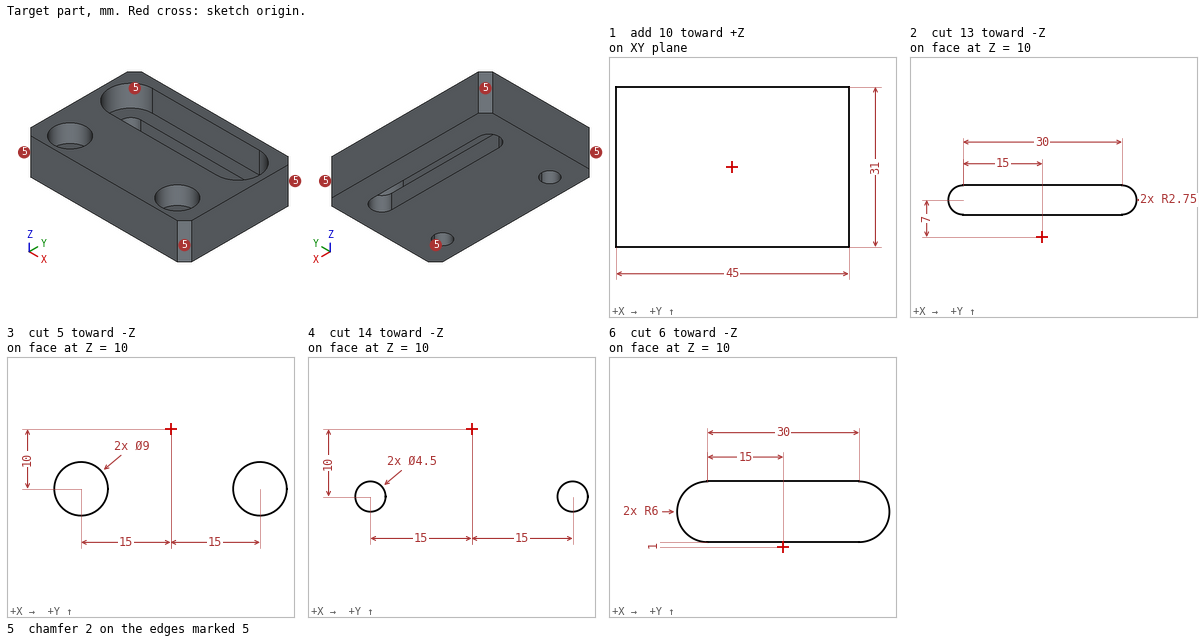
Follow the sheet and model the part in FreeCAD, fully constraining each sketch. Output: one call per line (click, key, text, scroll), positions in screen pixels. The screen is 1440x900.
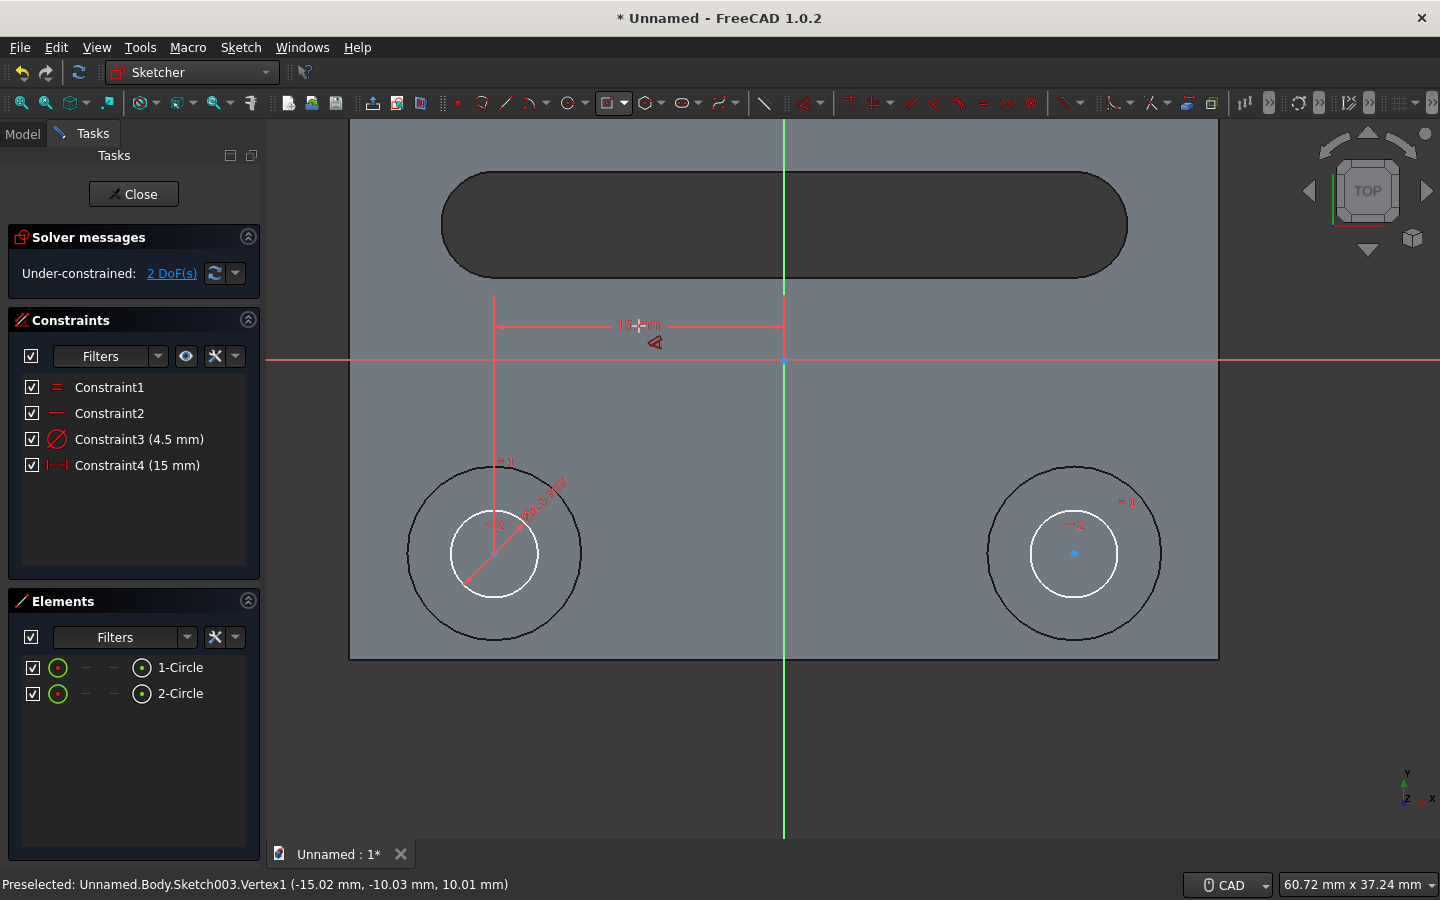
click(494, 554)
click(460, 457)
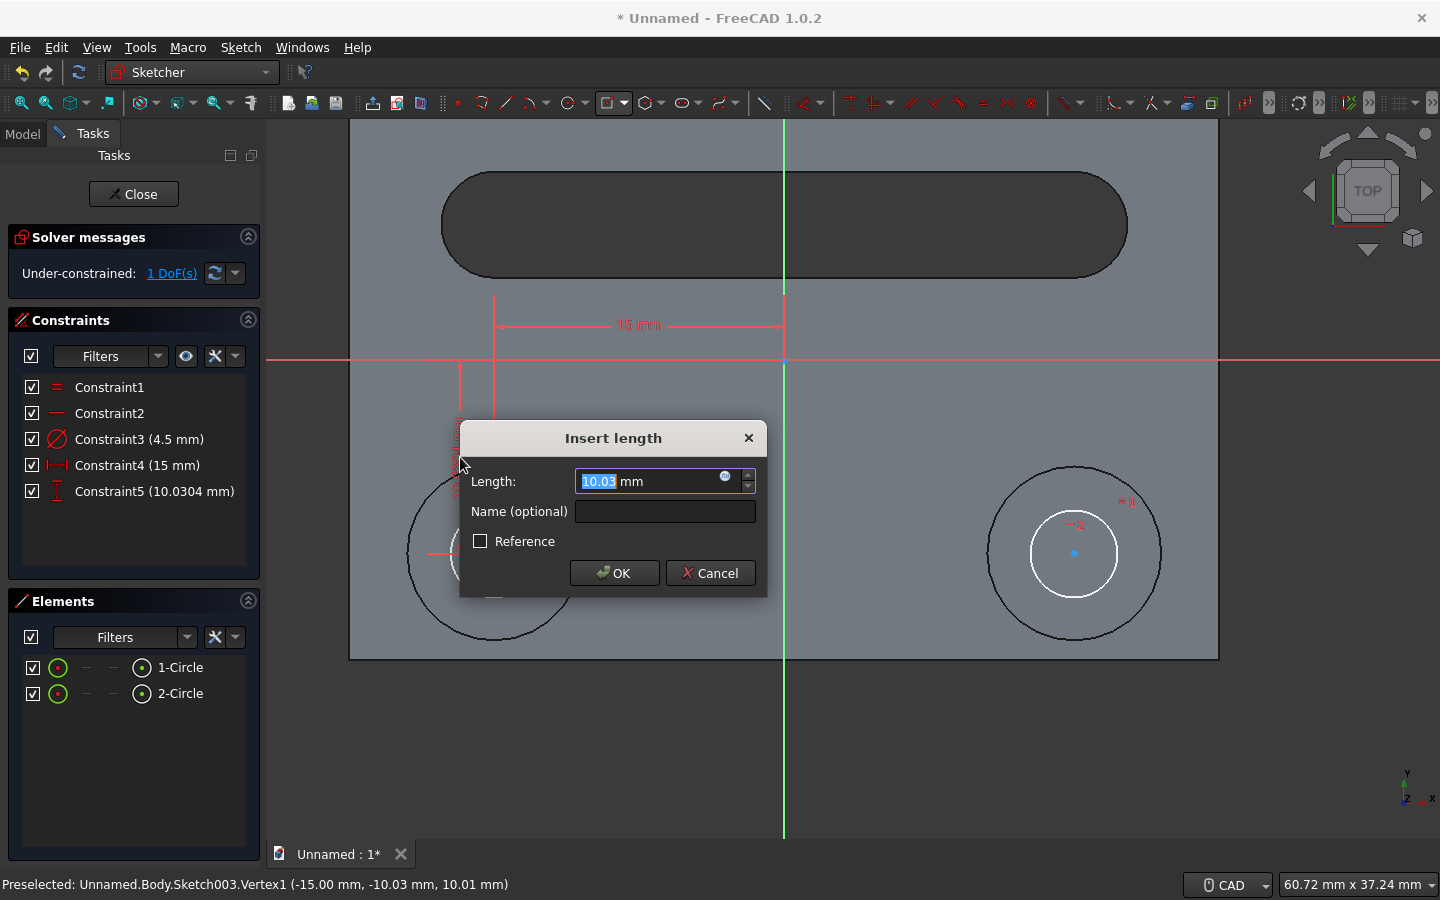
text(10)
key(Return)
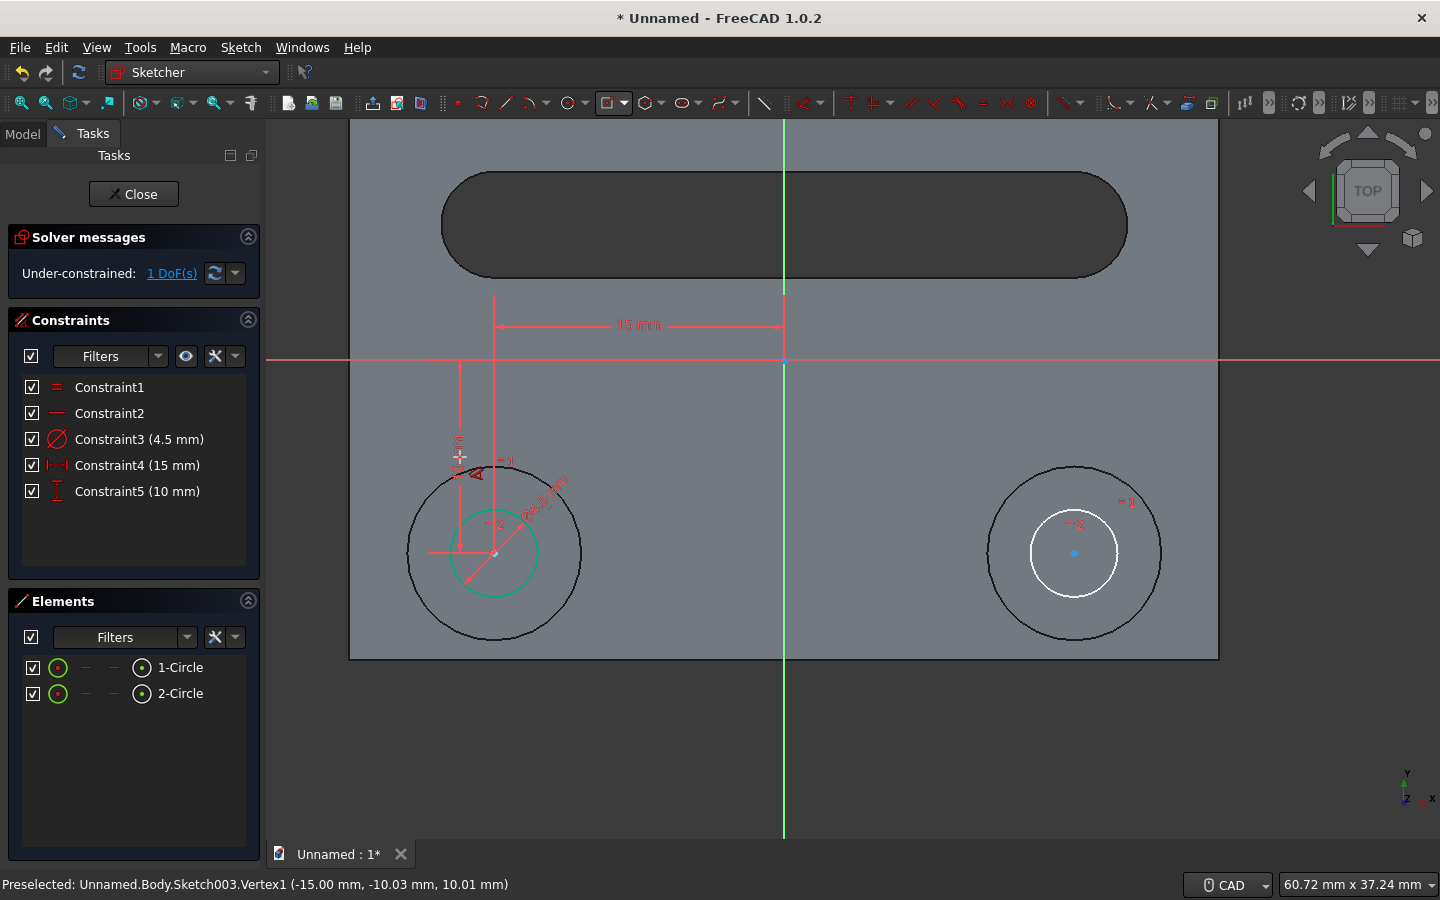
click(1074, 553)
click(929, 326)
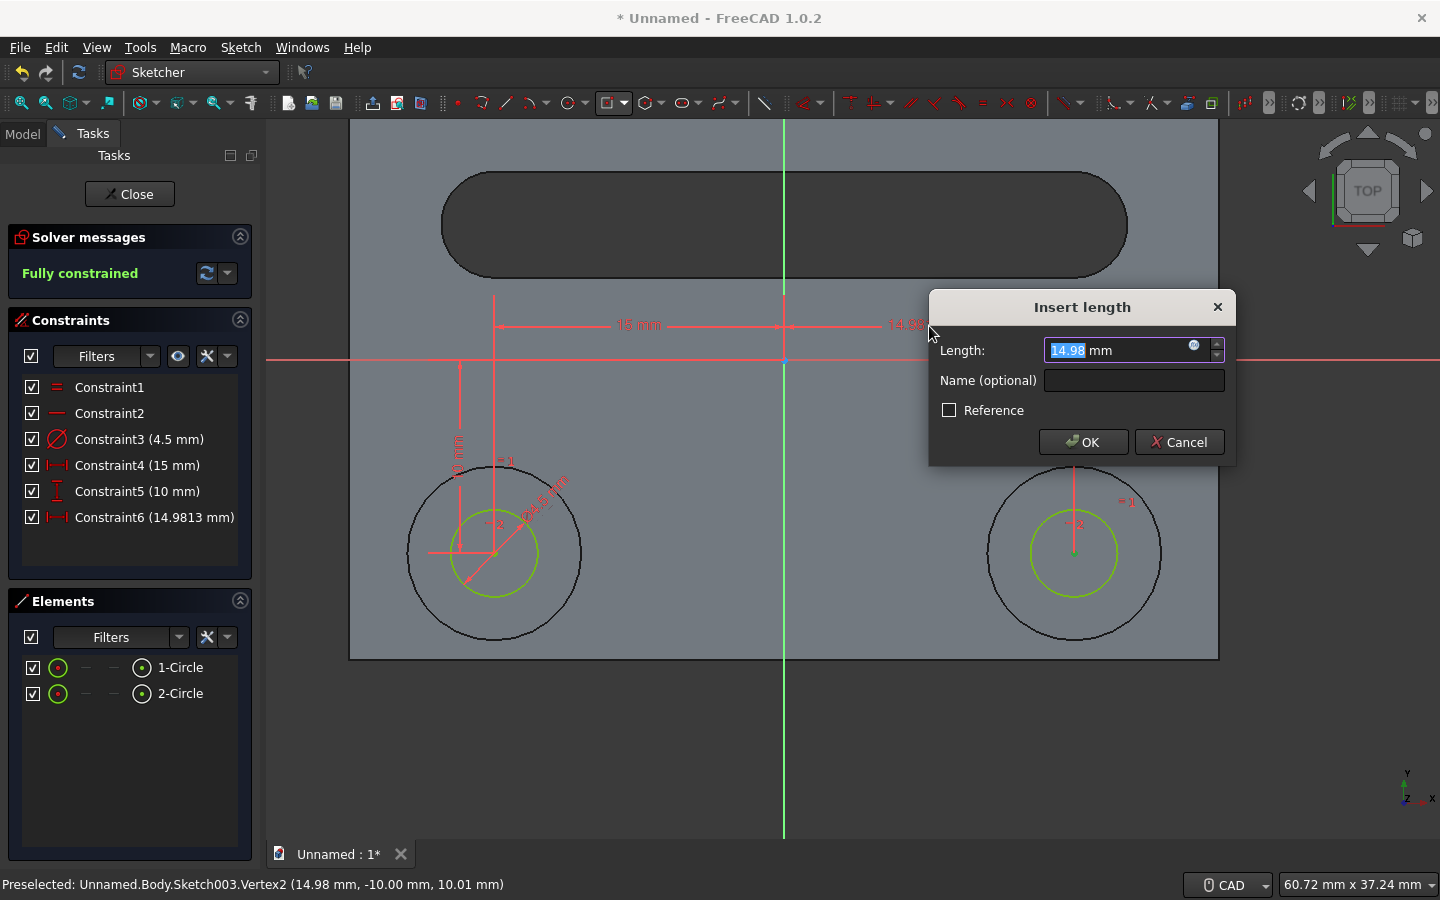
text(15)
key(Return)
key(Escape)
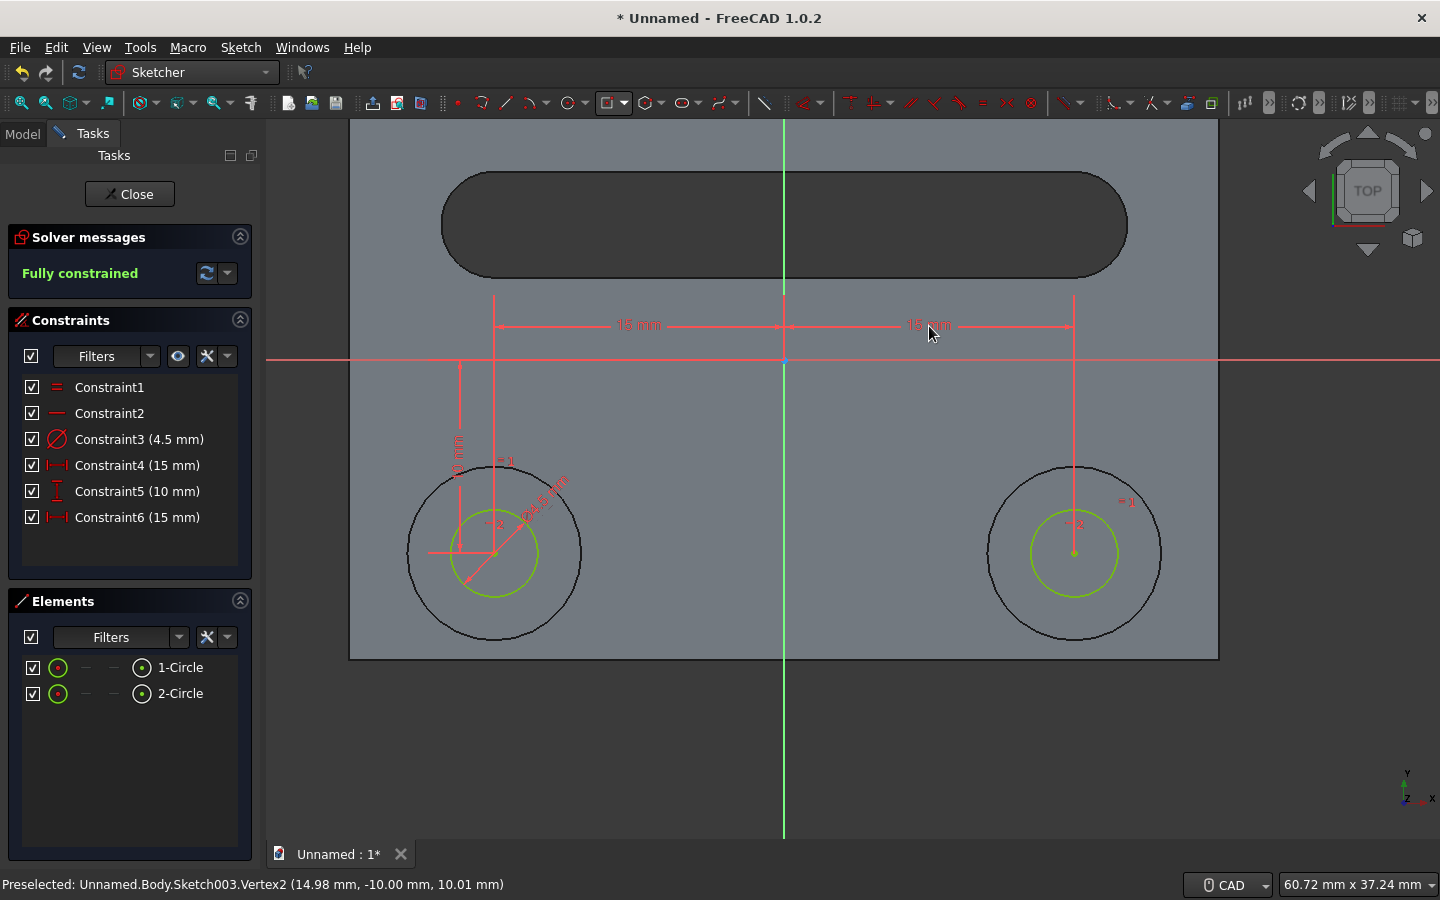
click(130, 194)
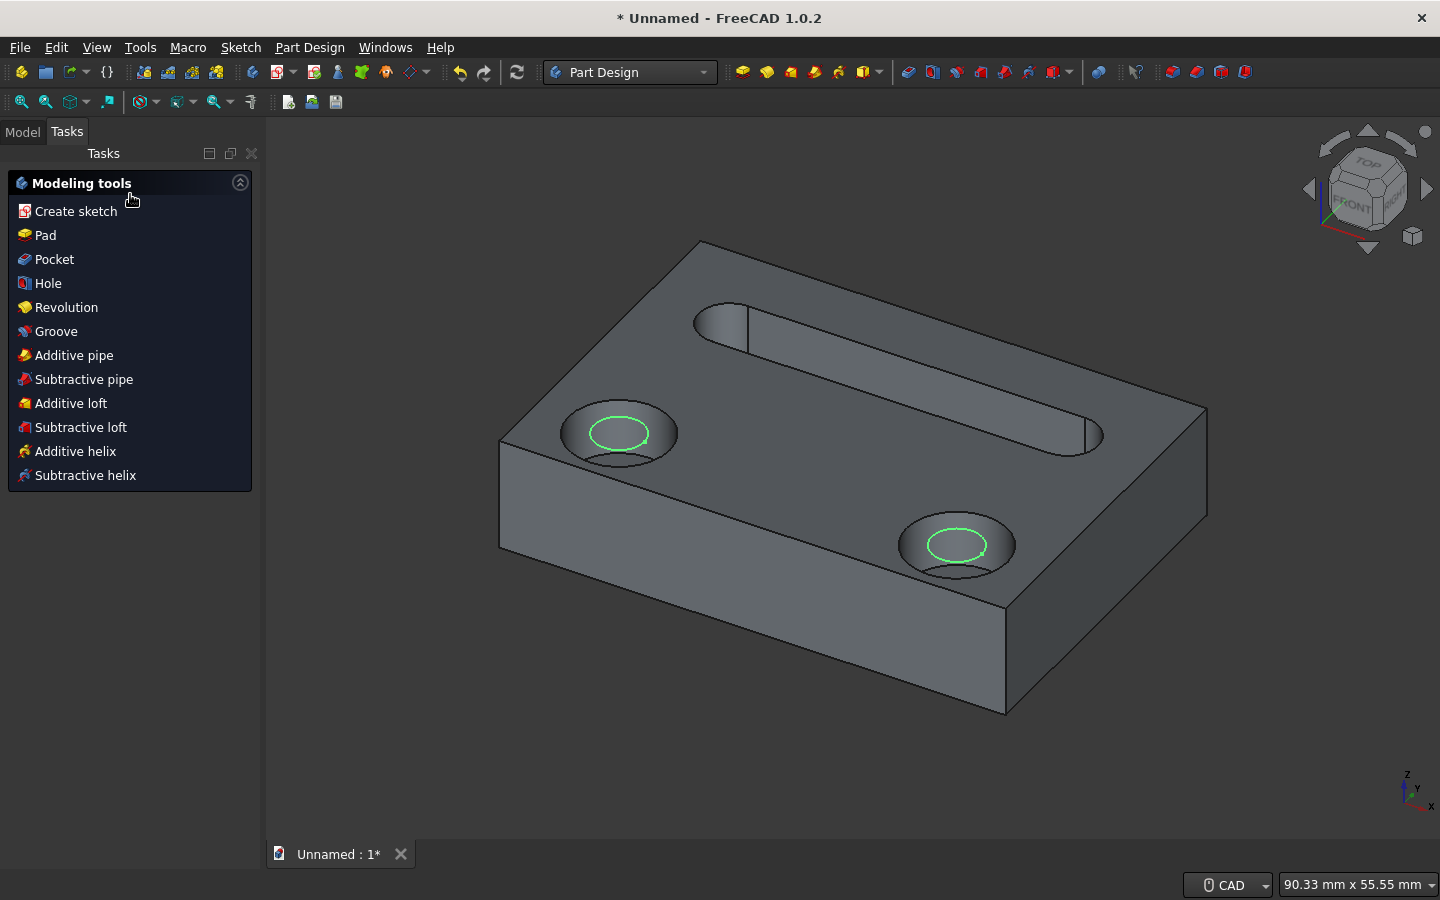
click(910, 72)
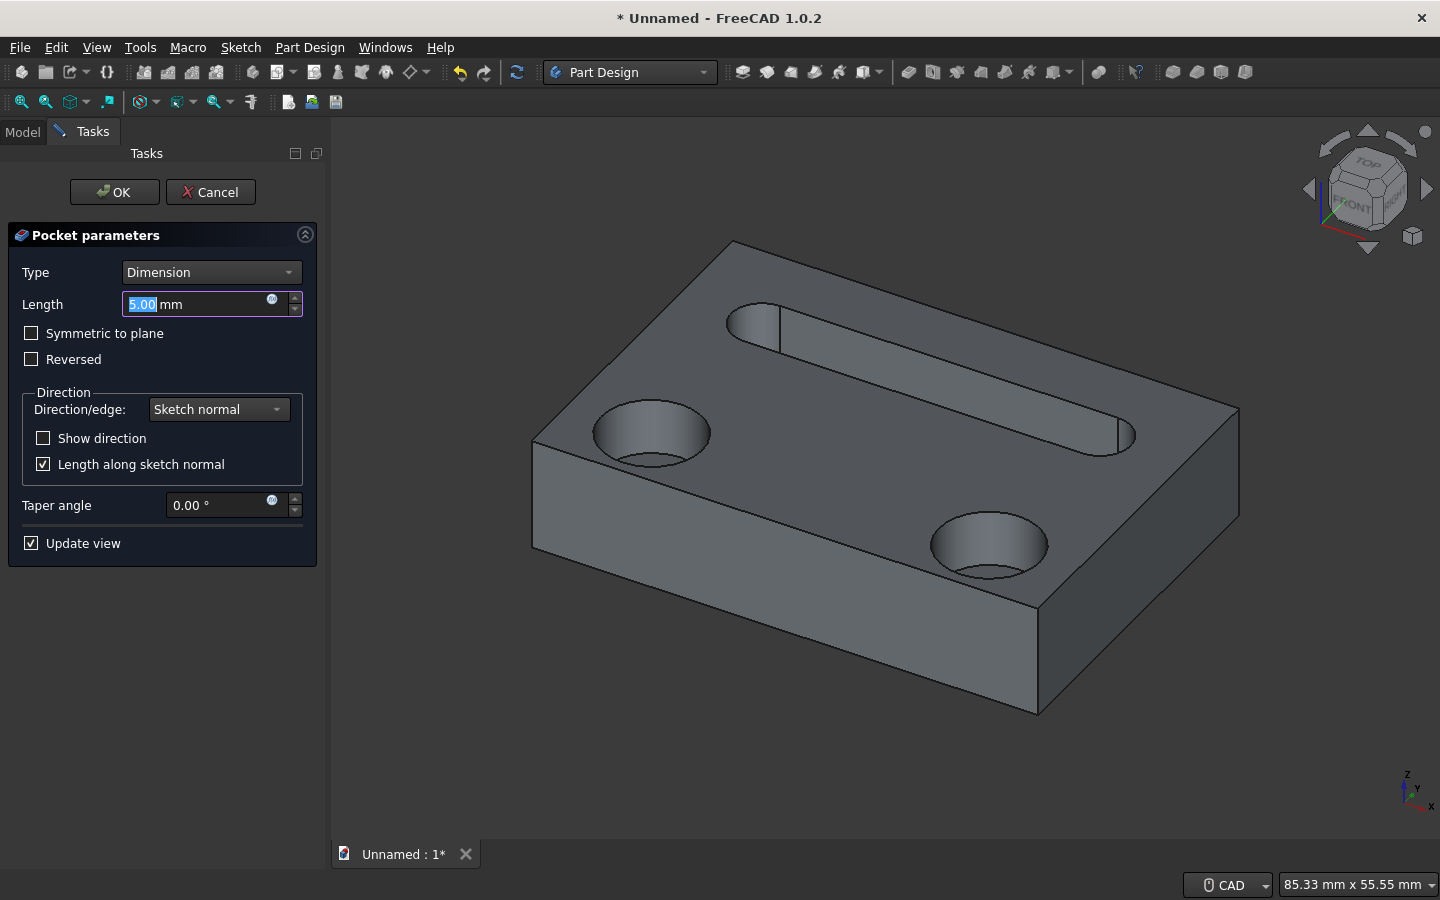
text(14)
key(Tab)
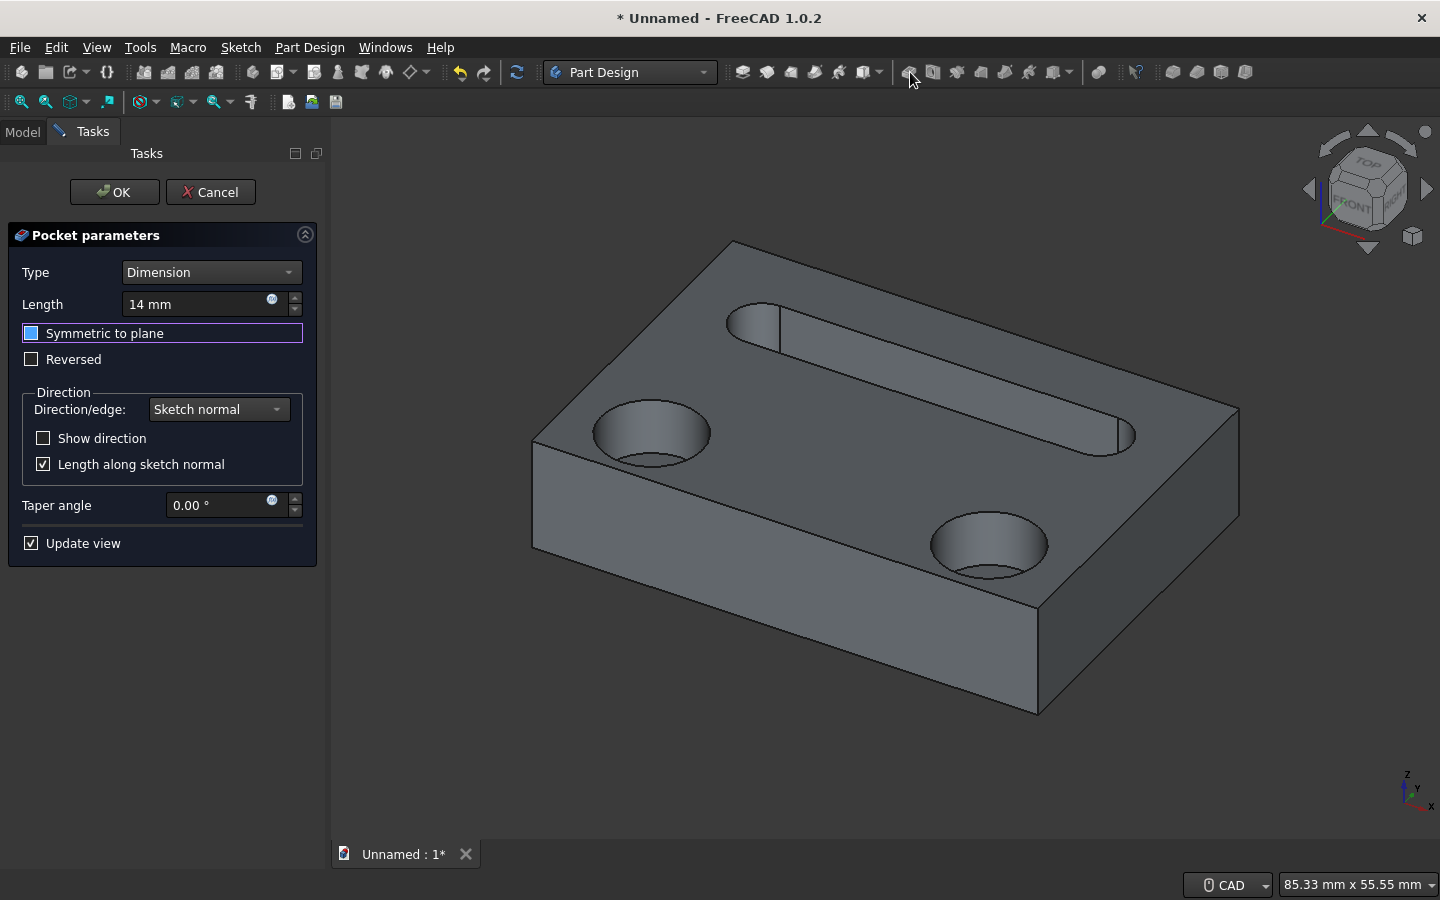
click(115, 192)